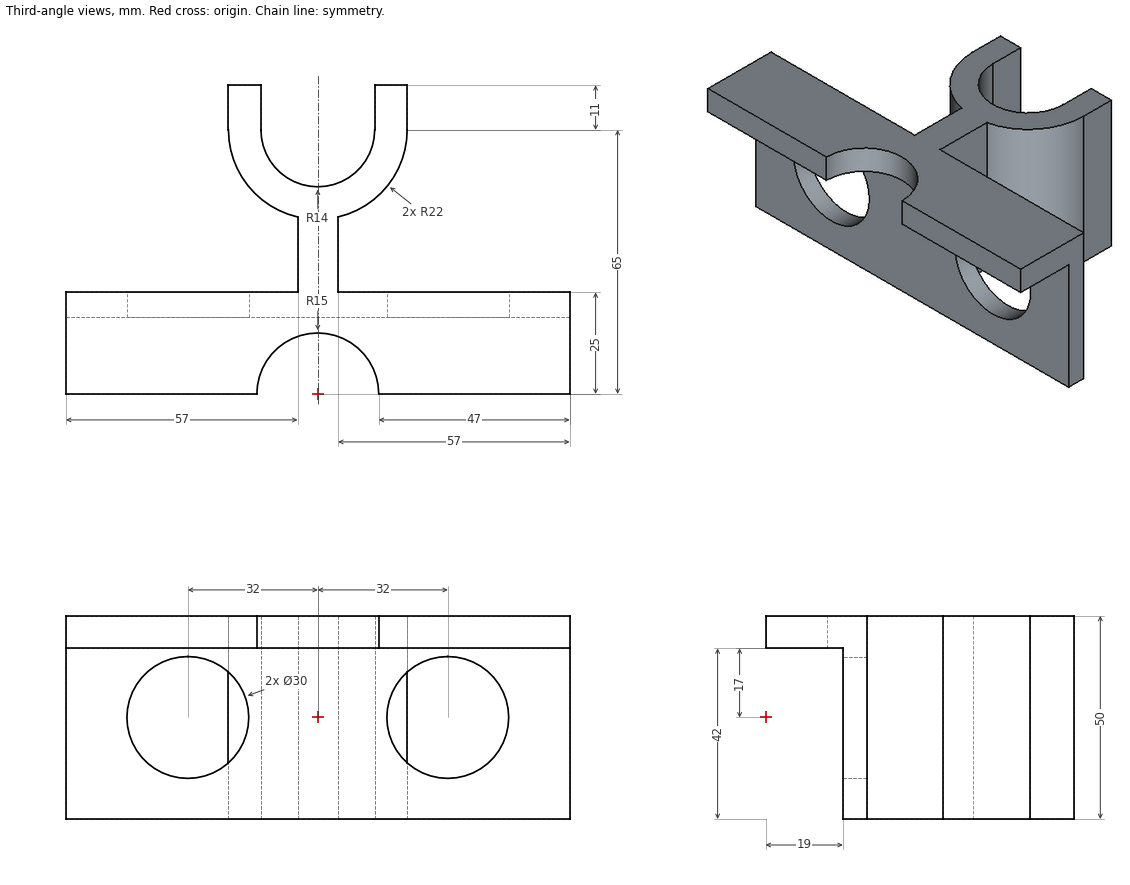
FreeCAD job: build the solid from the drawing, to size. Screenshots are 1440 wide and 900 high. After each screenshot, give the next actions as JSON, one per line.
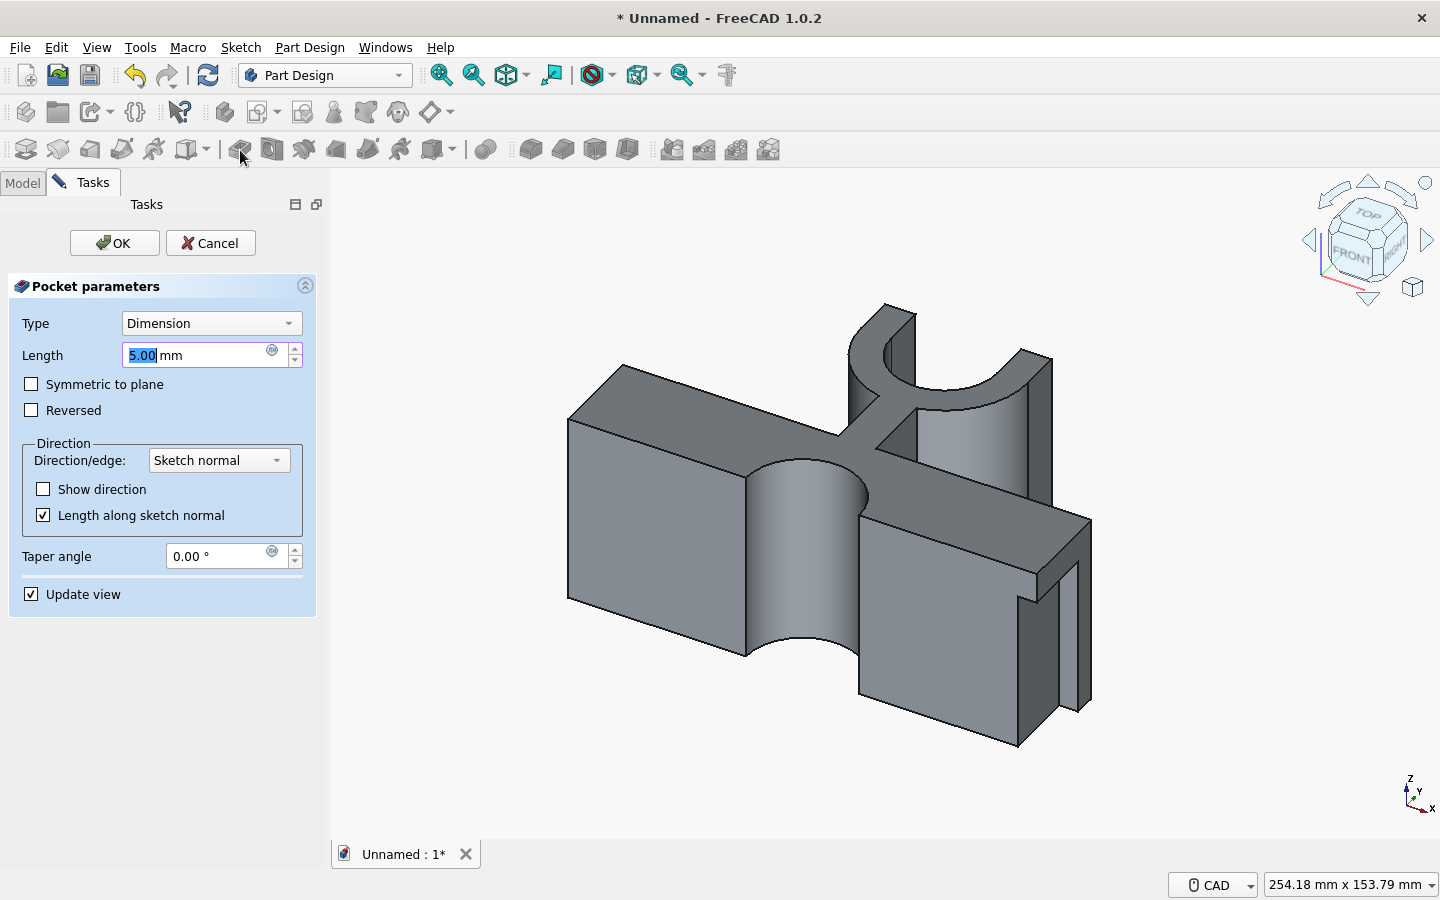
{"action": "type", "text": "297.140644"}
{"action": "key", "text": "Tab"}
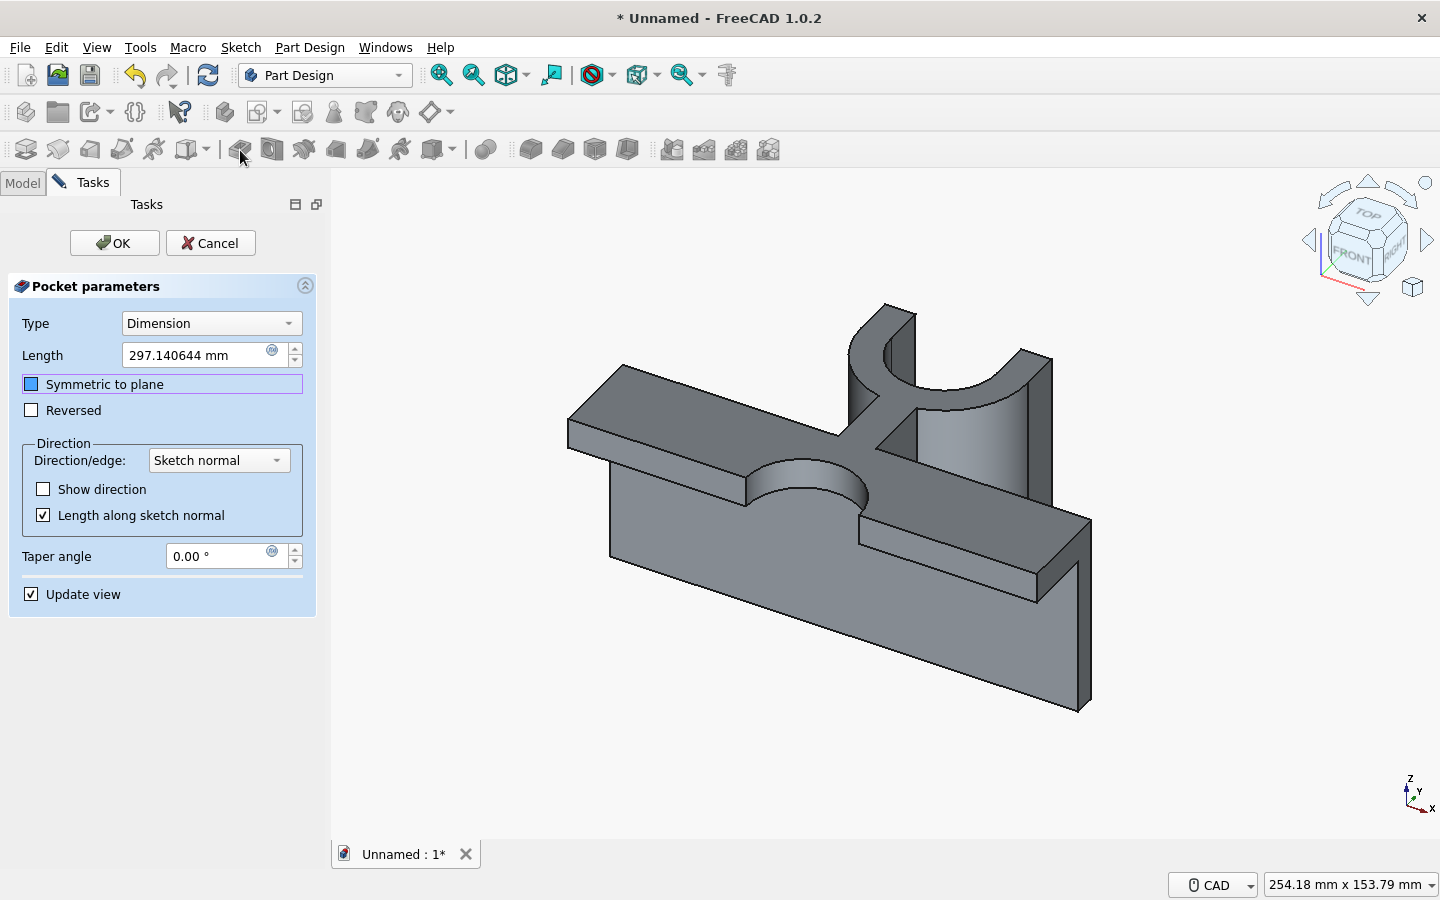
{"action": "left_click", "coordinate": [30, 384]}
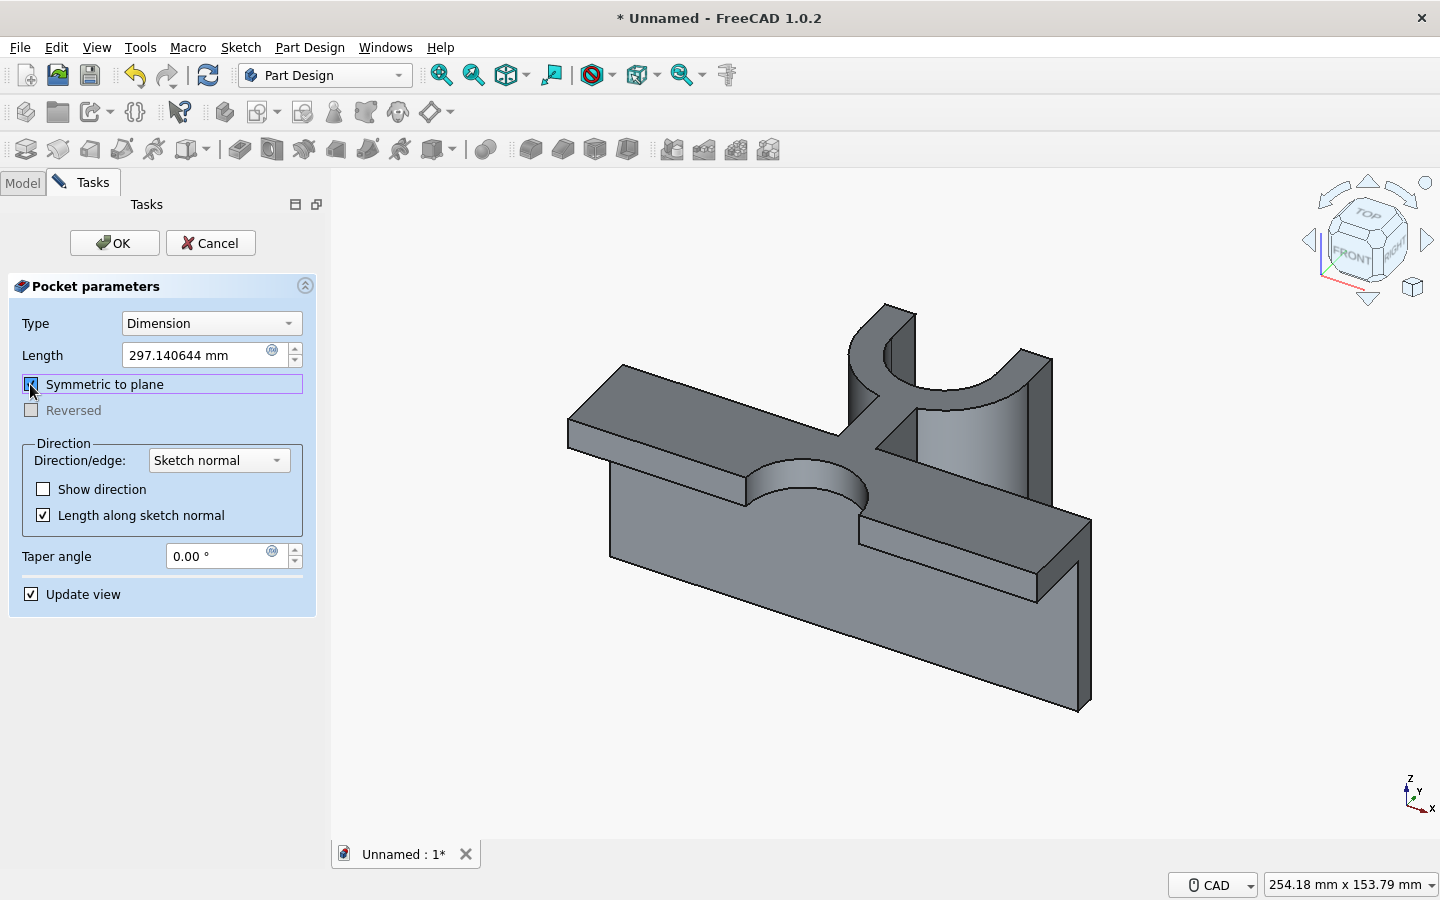
{"action": "left_click", "coordinate": [115, 243]}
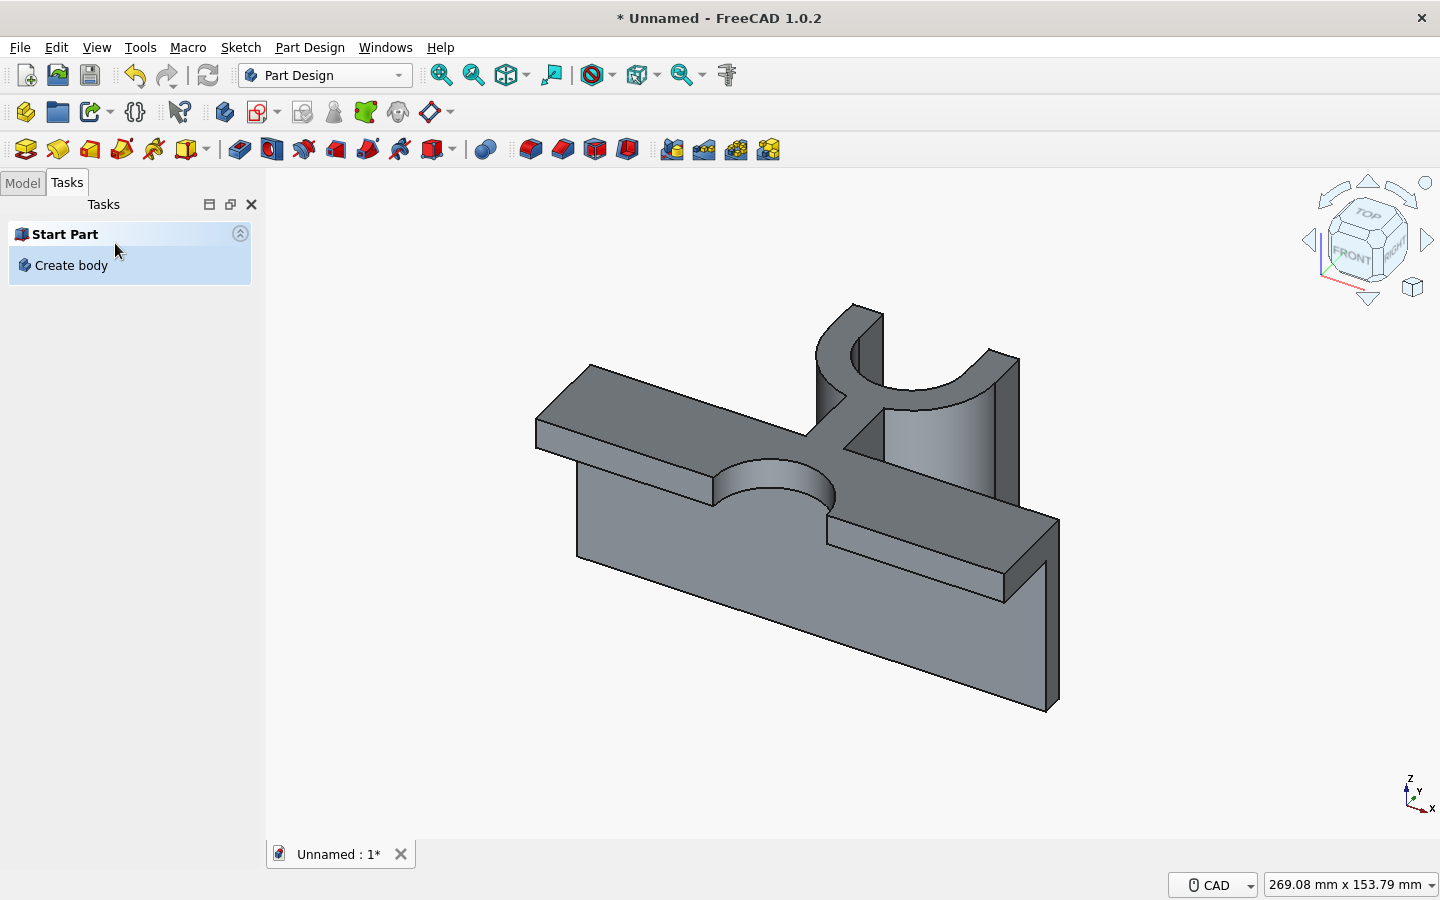
{"action": "key", "text": "4"}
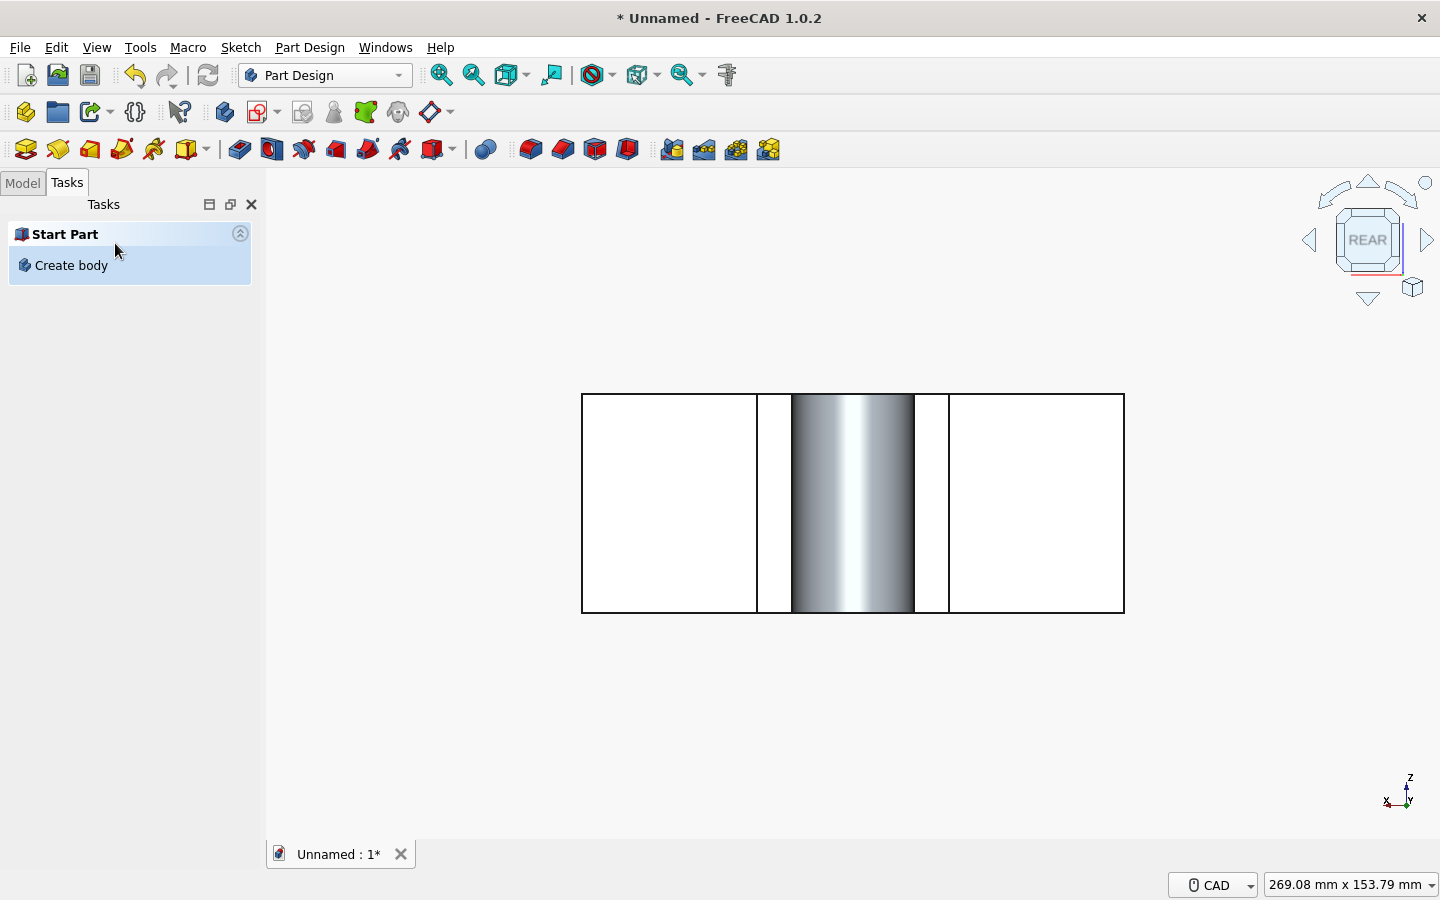
{"action": "left_click", "coordinate": [999, 502]}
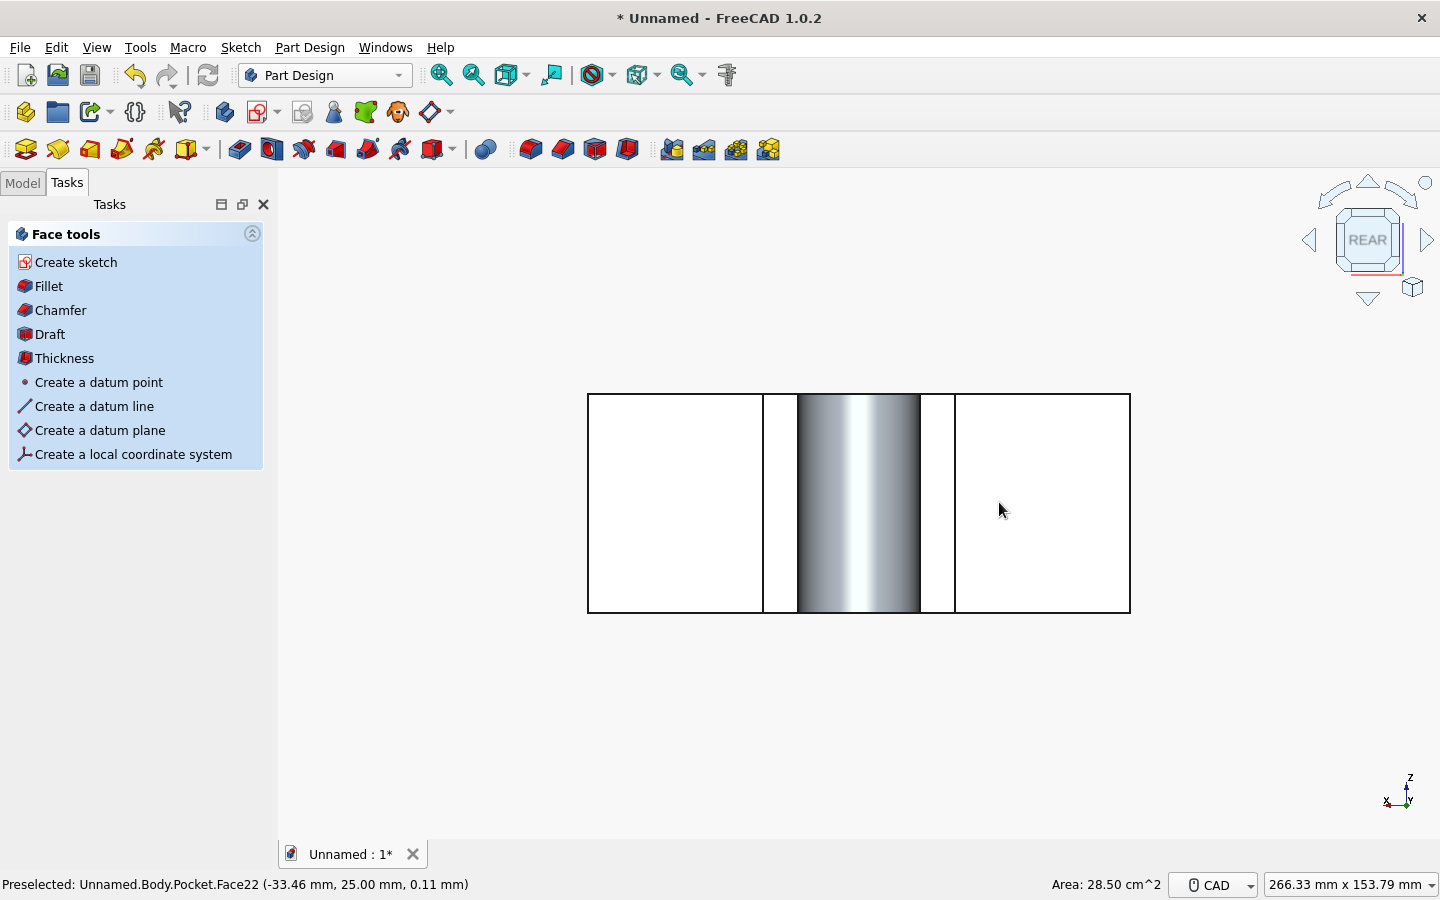
{"action": "left_click", "coordinate": [258, 112]}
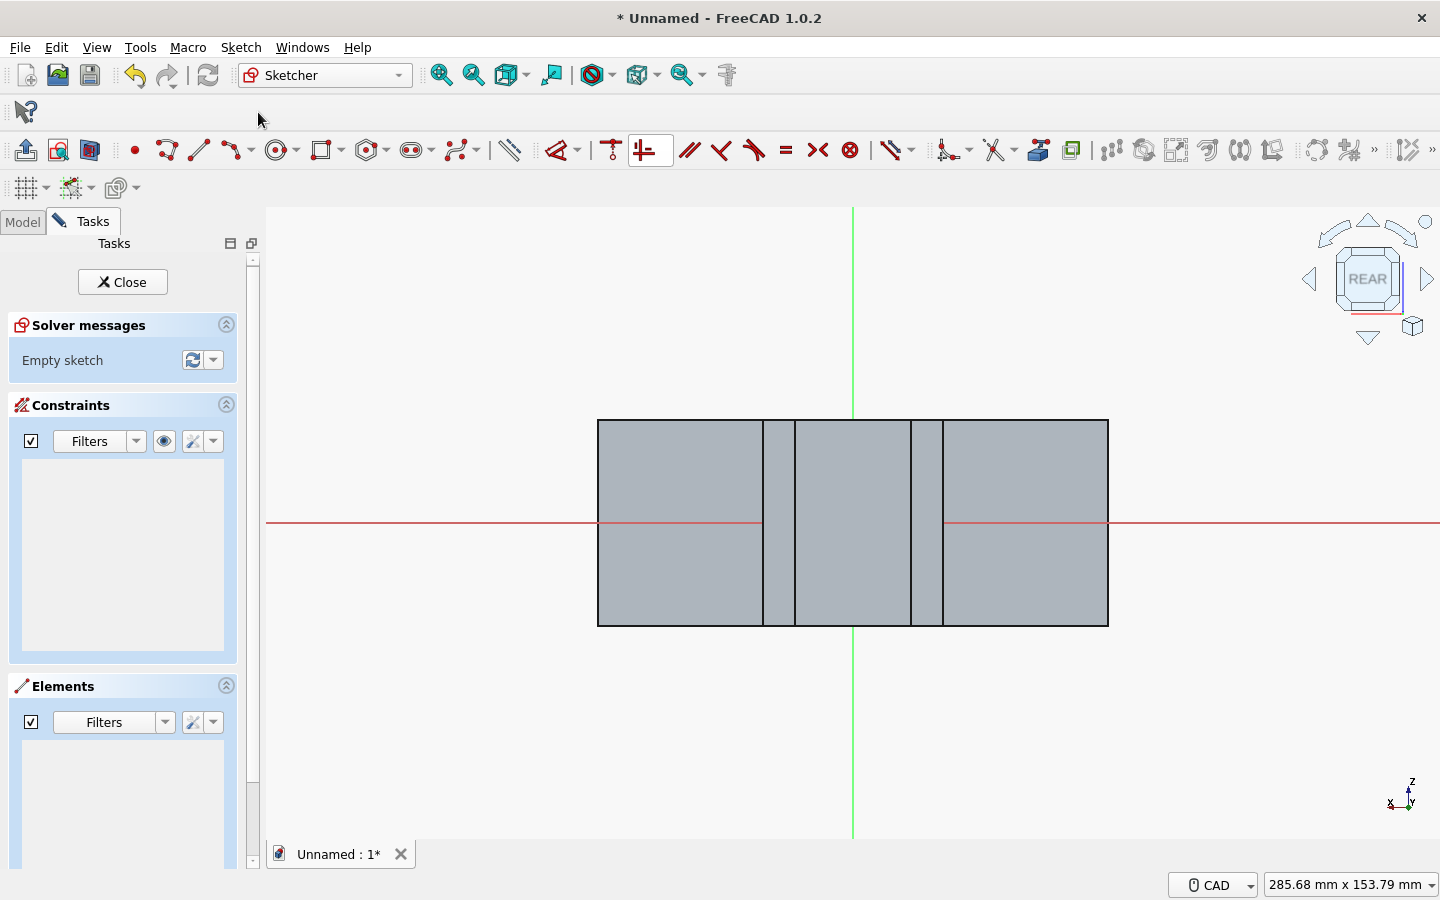
{"action": "left_click", "coordinate": [90, 150]}